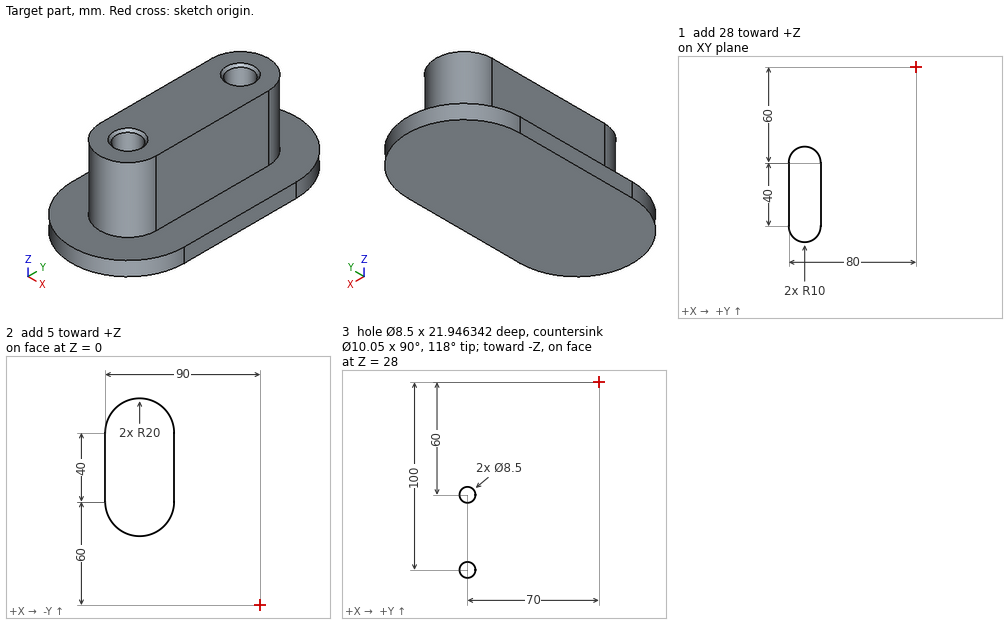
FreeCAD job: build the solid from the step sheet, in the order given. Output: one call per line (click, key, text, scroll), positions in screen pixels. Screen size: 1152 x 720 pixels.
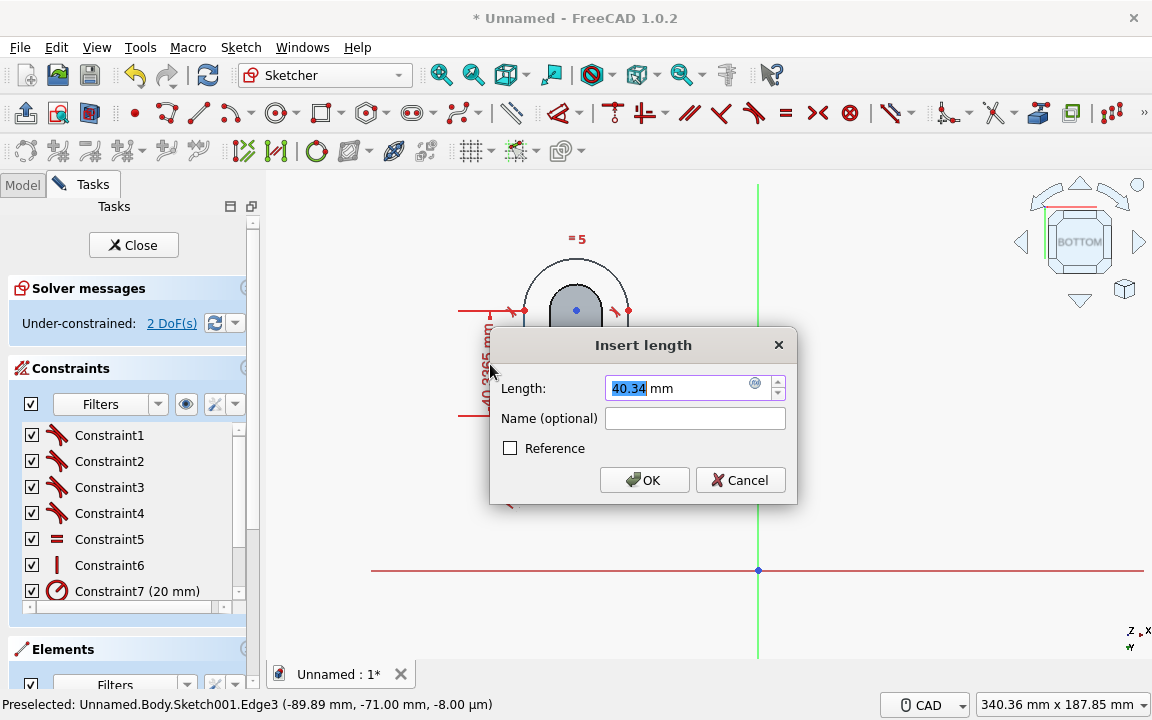
text(40)
key(Return)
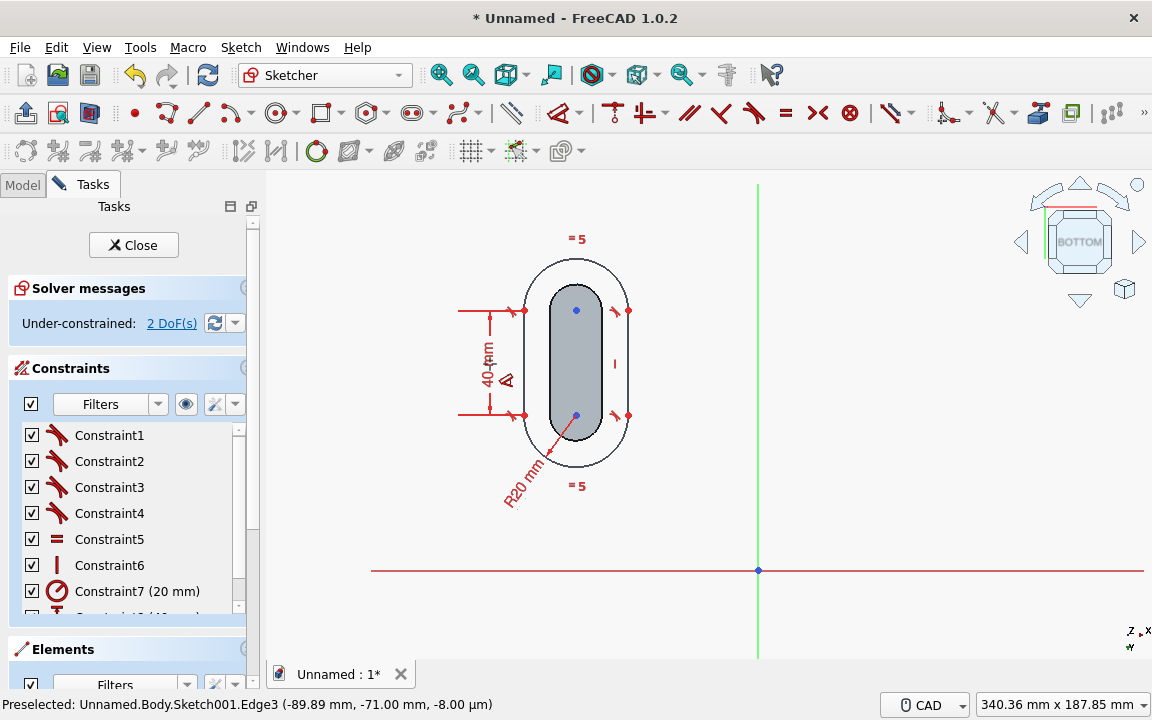
click(524, 415)
click(641, 605)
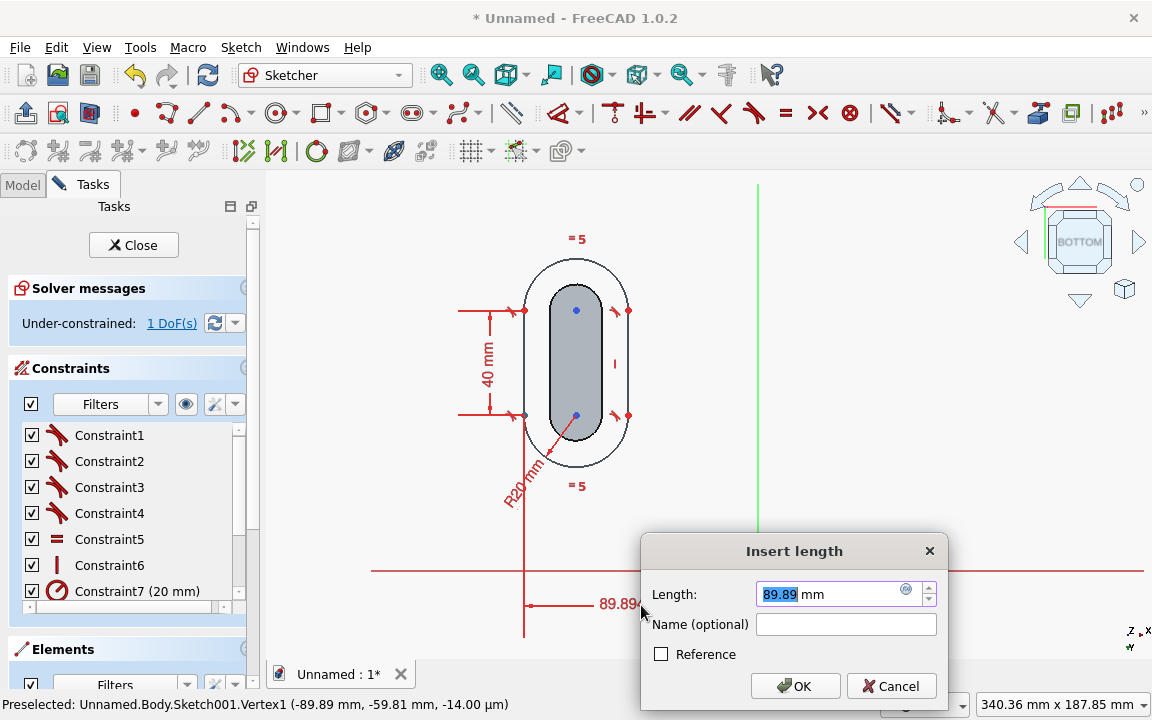
text(90)
key(Return)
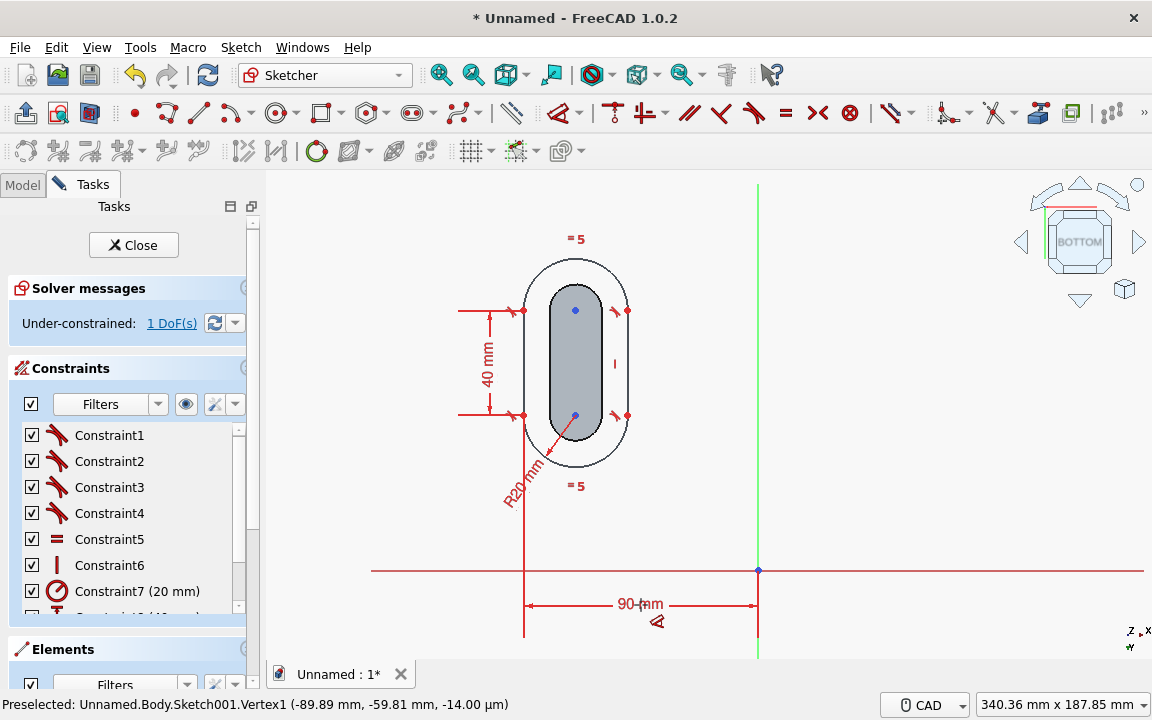
click(524, 415)
click(792, 493)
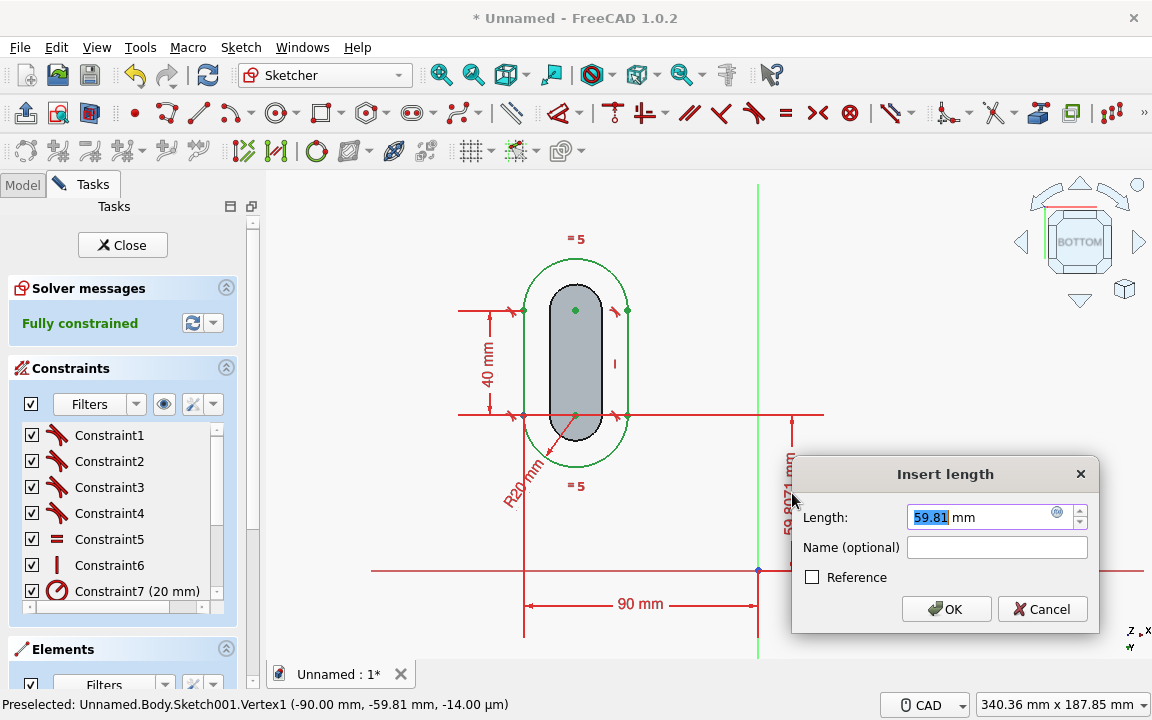
text(60)
key(Return)
key(Escape)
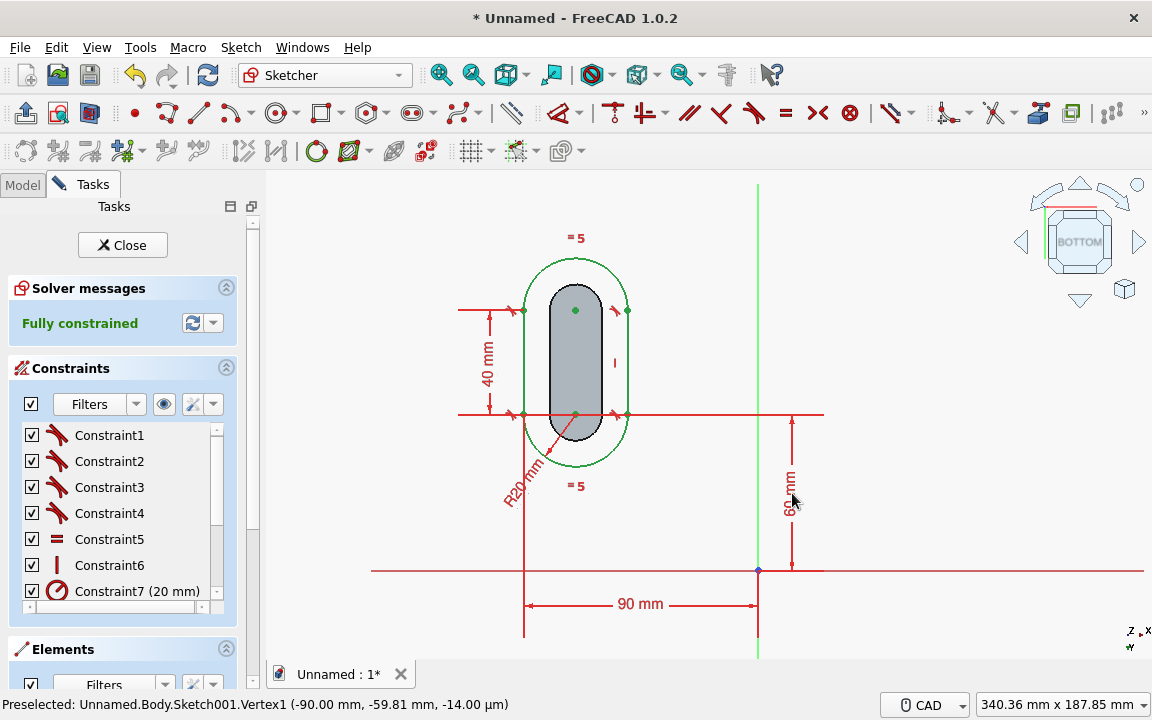
click(123, 245)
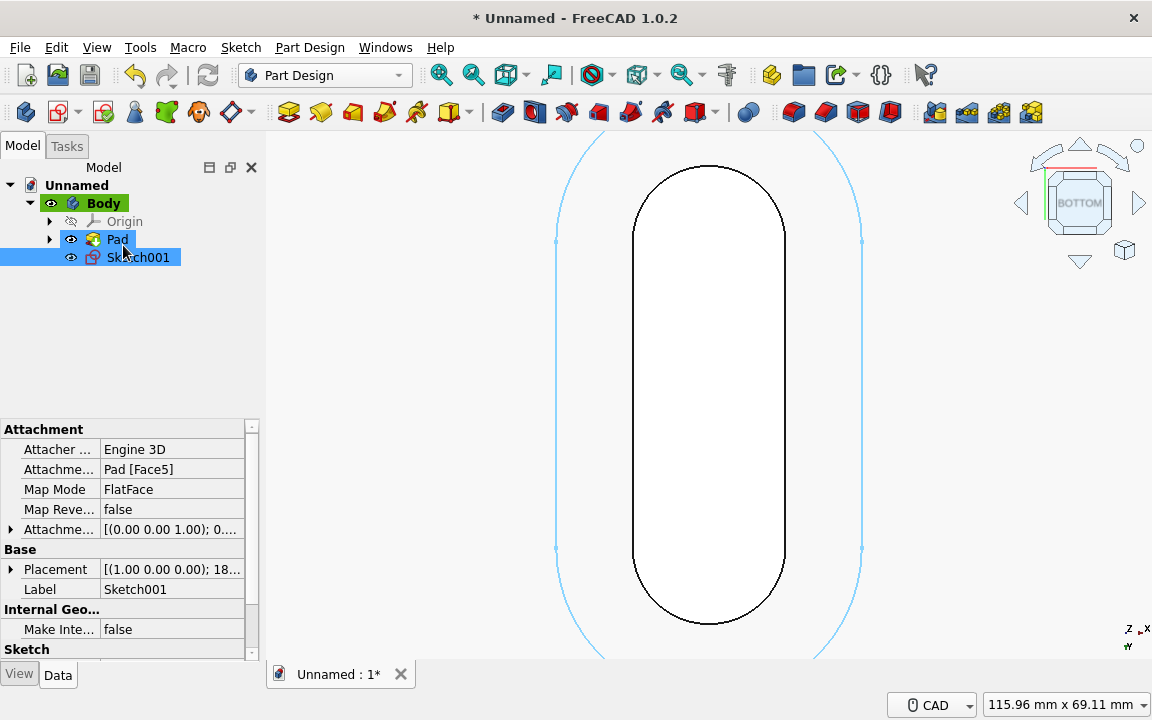
click(290, 112)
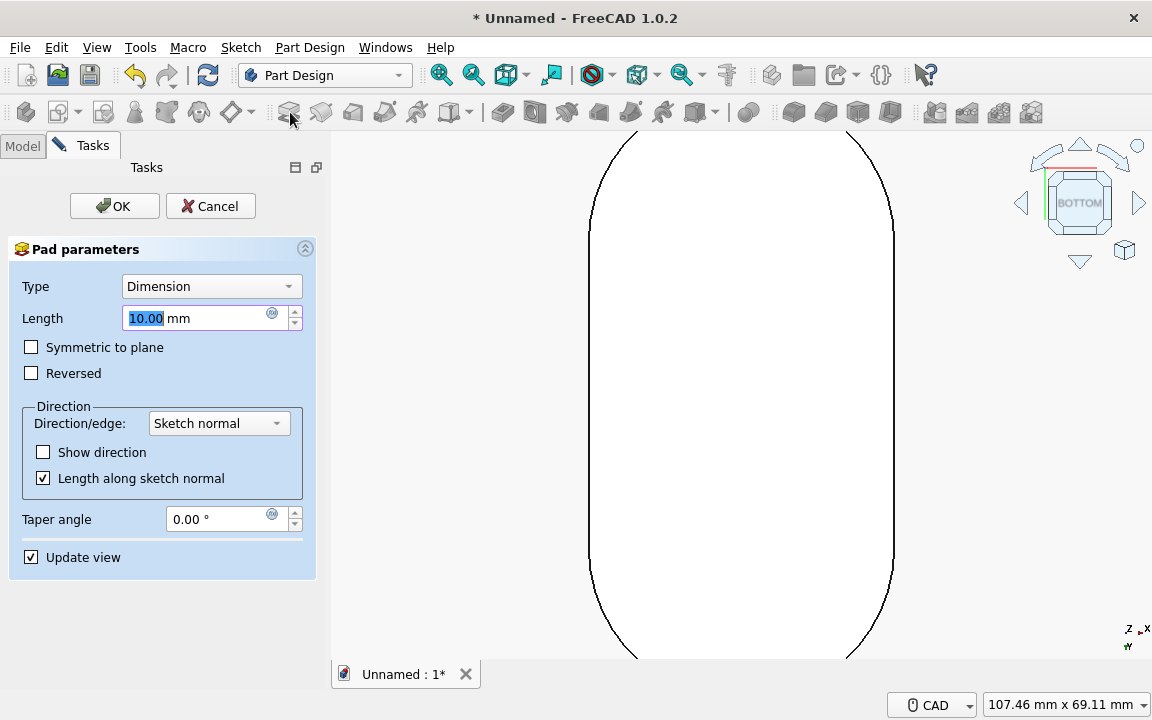
text(5)
key(Tab)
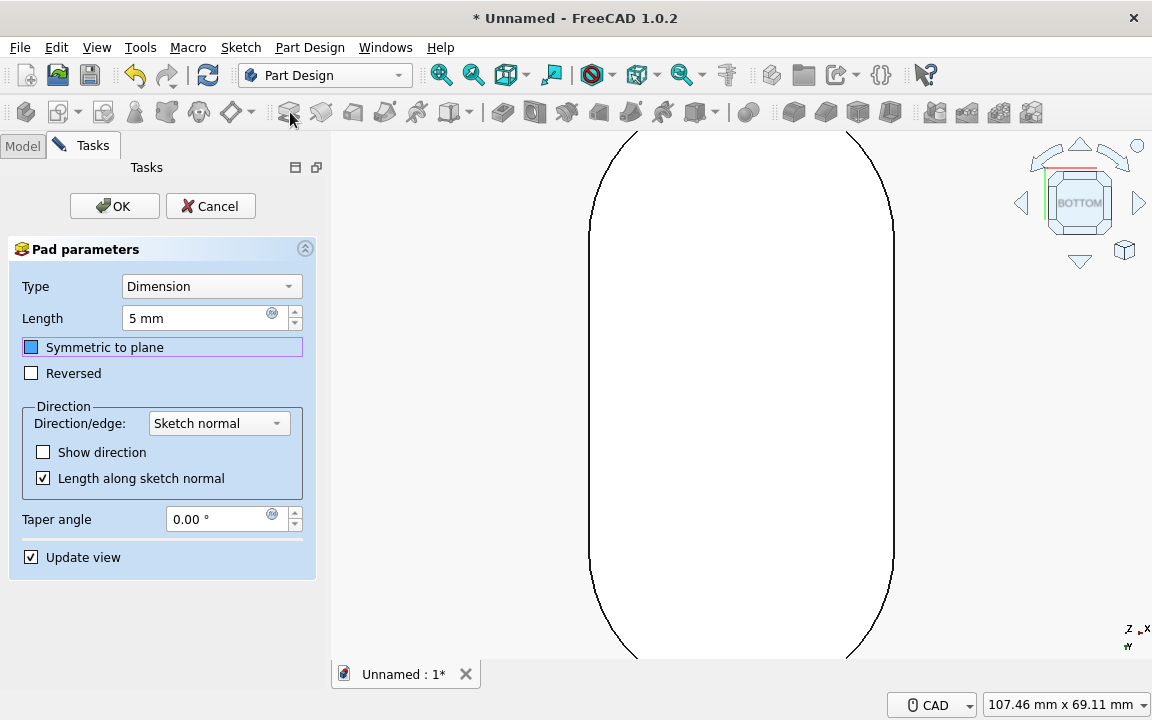
click(30, 373)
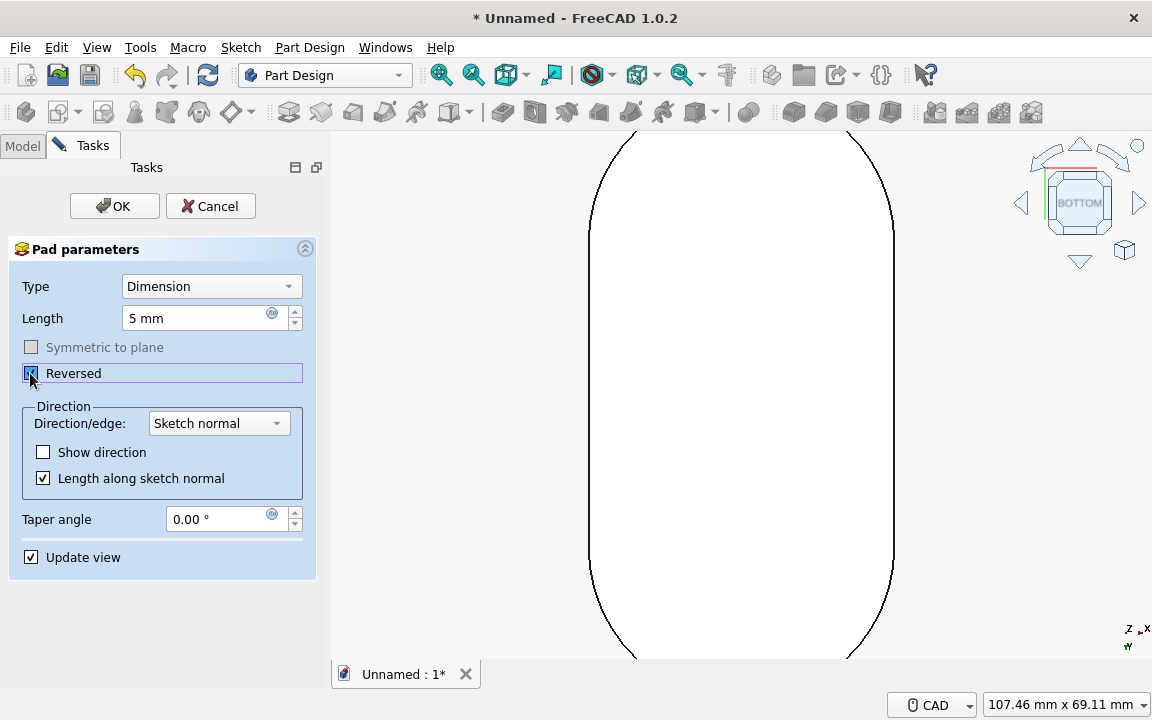
click(115, 206)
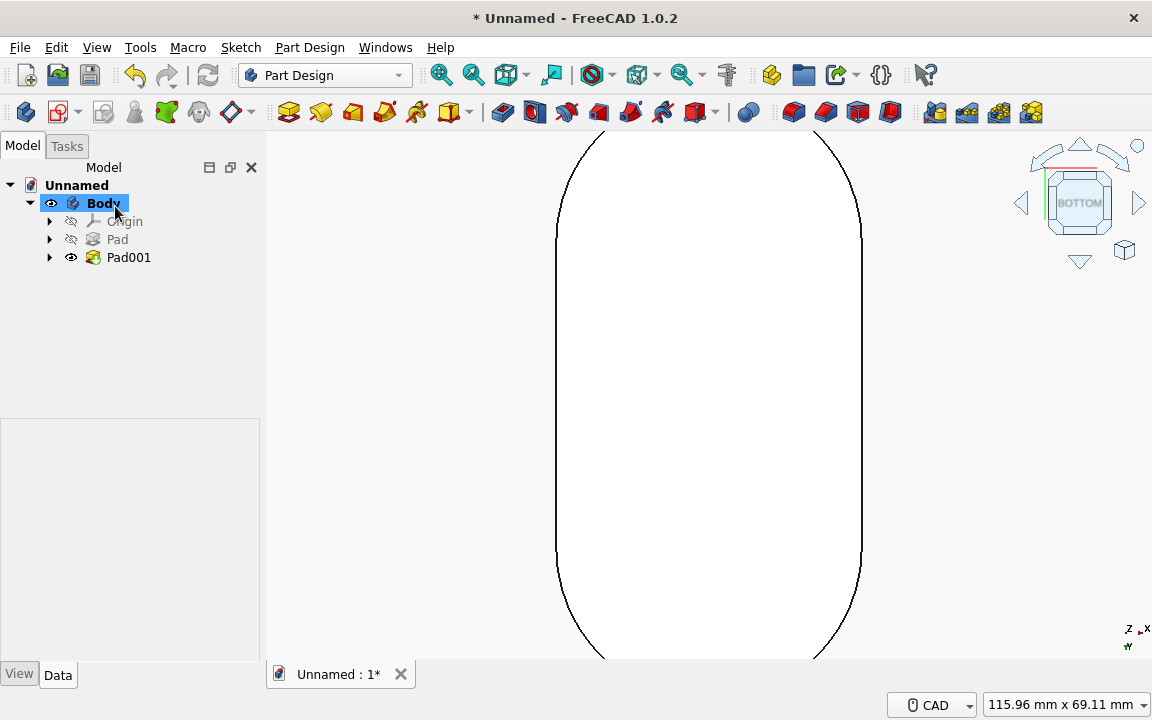
click(442, 76)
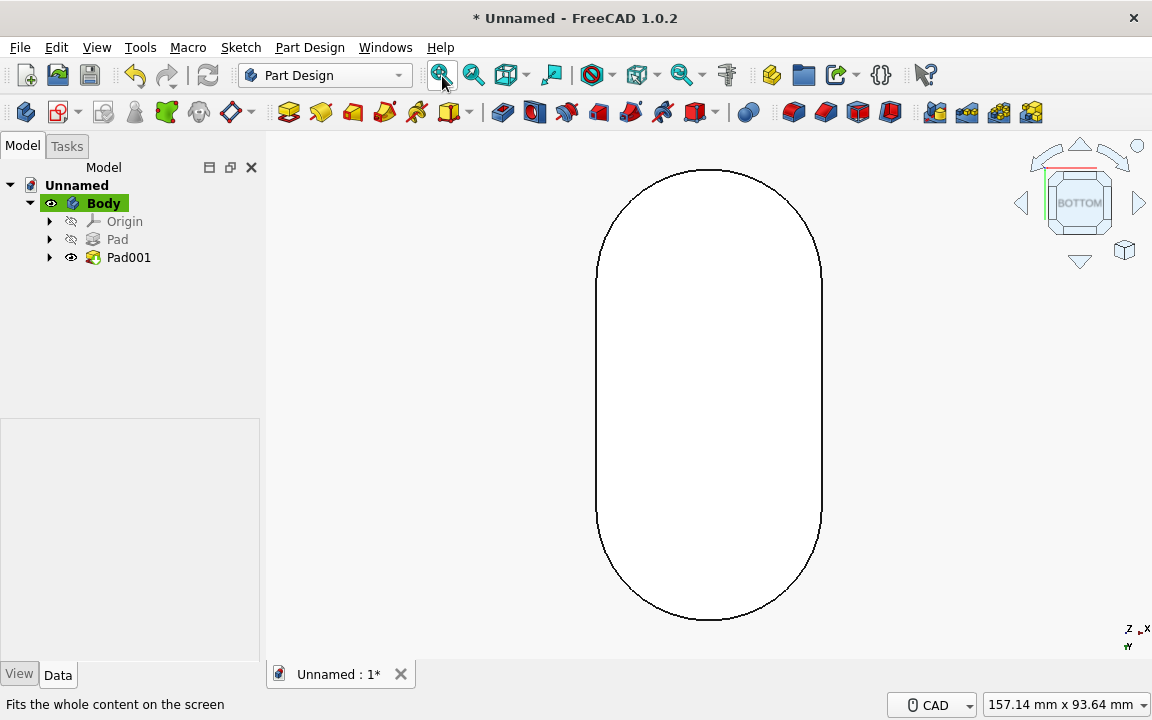
key(0)